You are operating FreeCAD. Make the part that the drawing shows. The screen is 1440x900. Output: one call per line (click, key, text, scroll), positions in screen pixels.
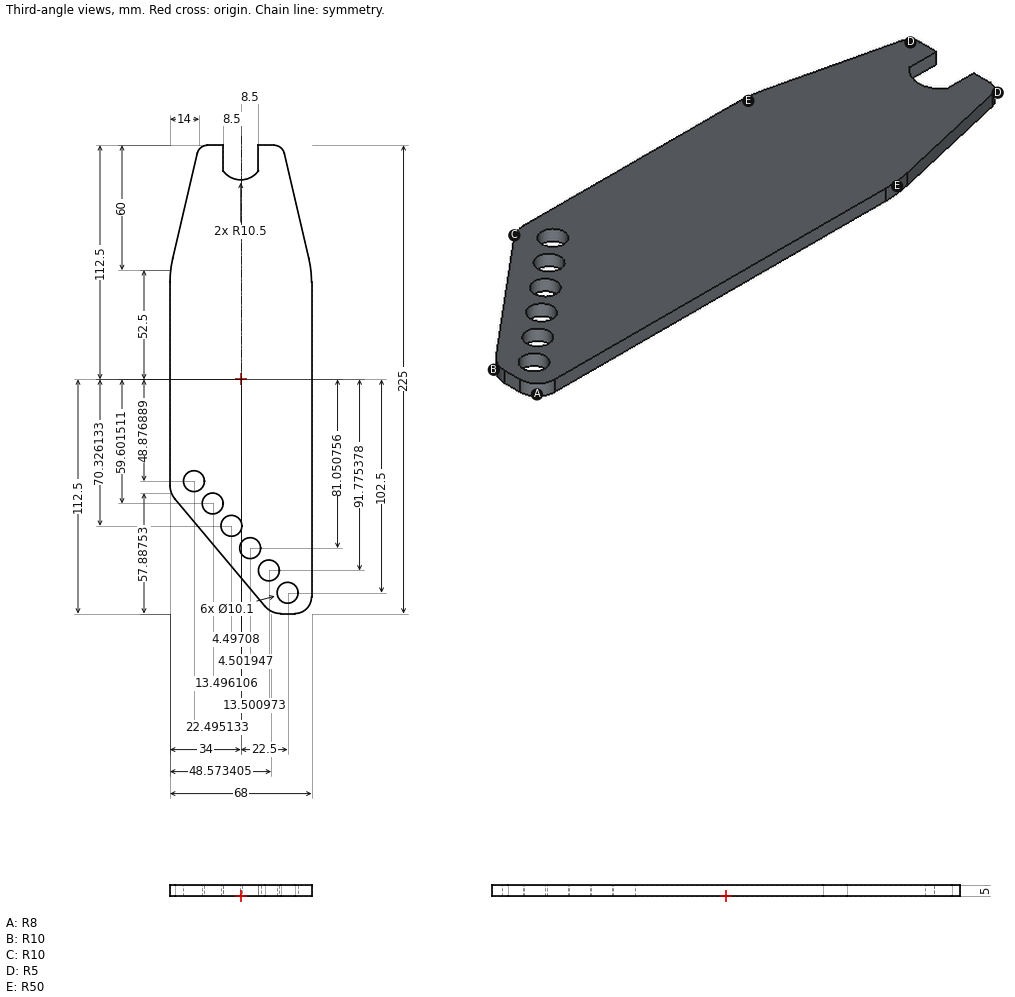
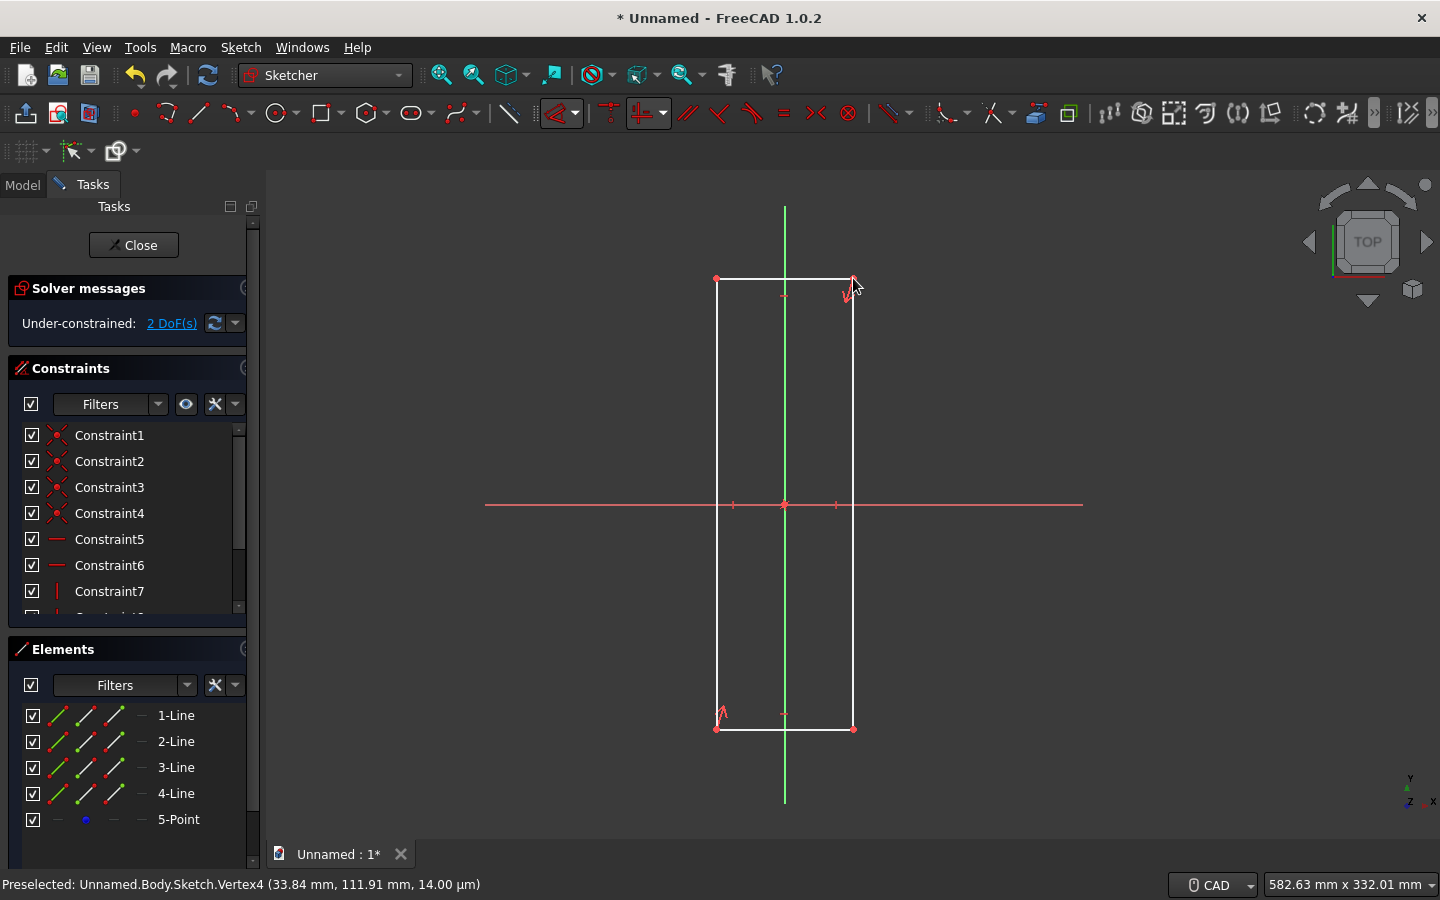
click(758, 730)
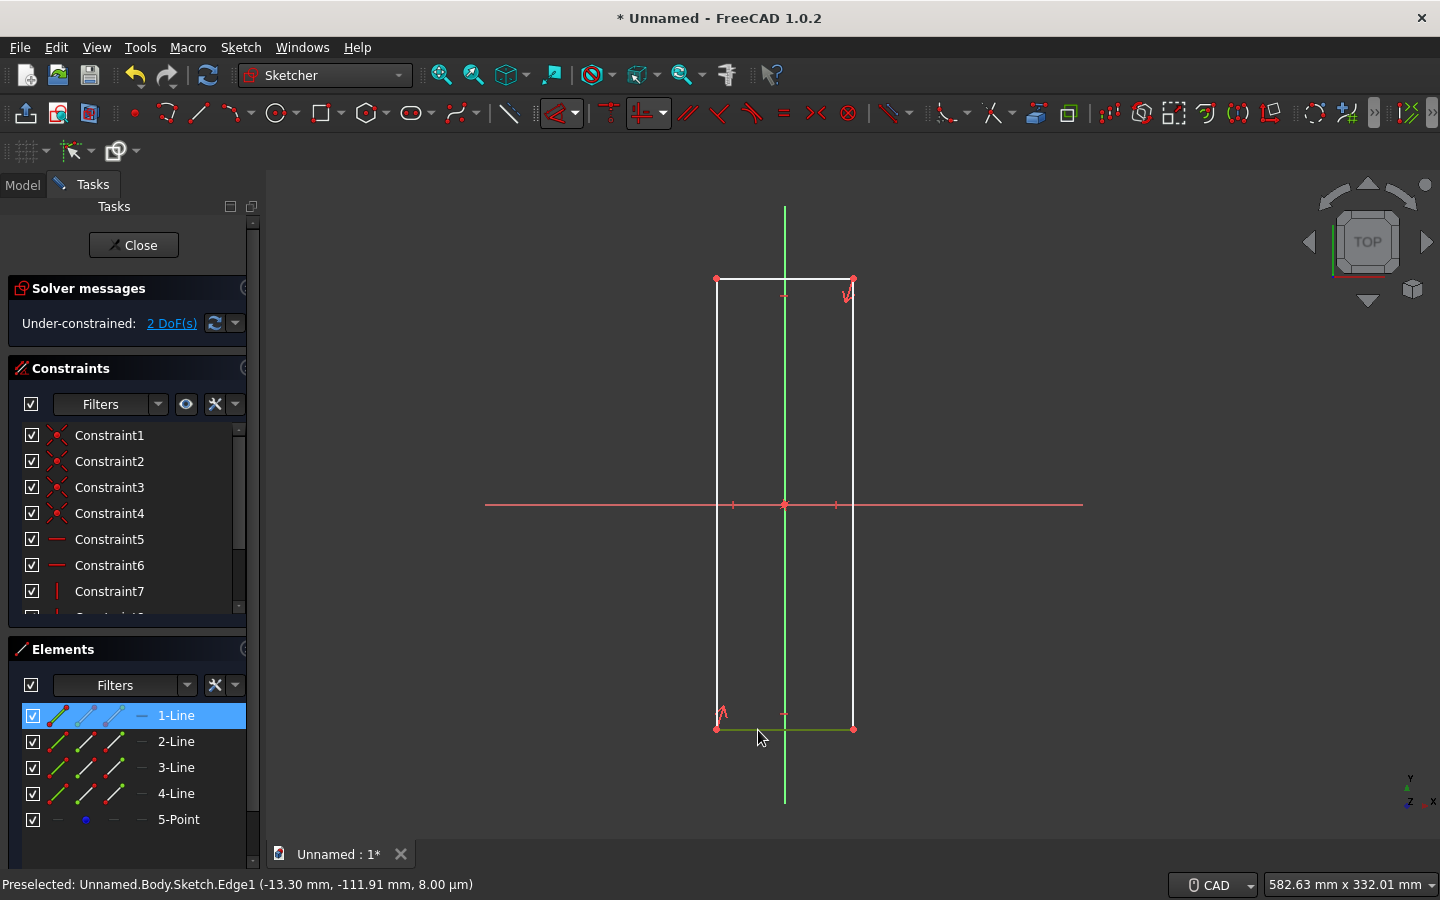
key(l)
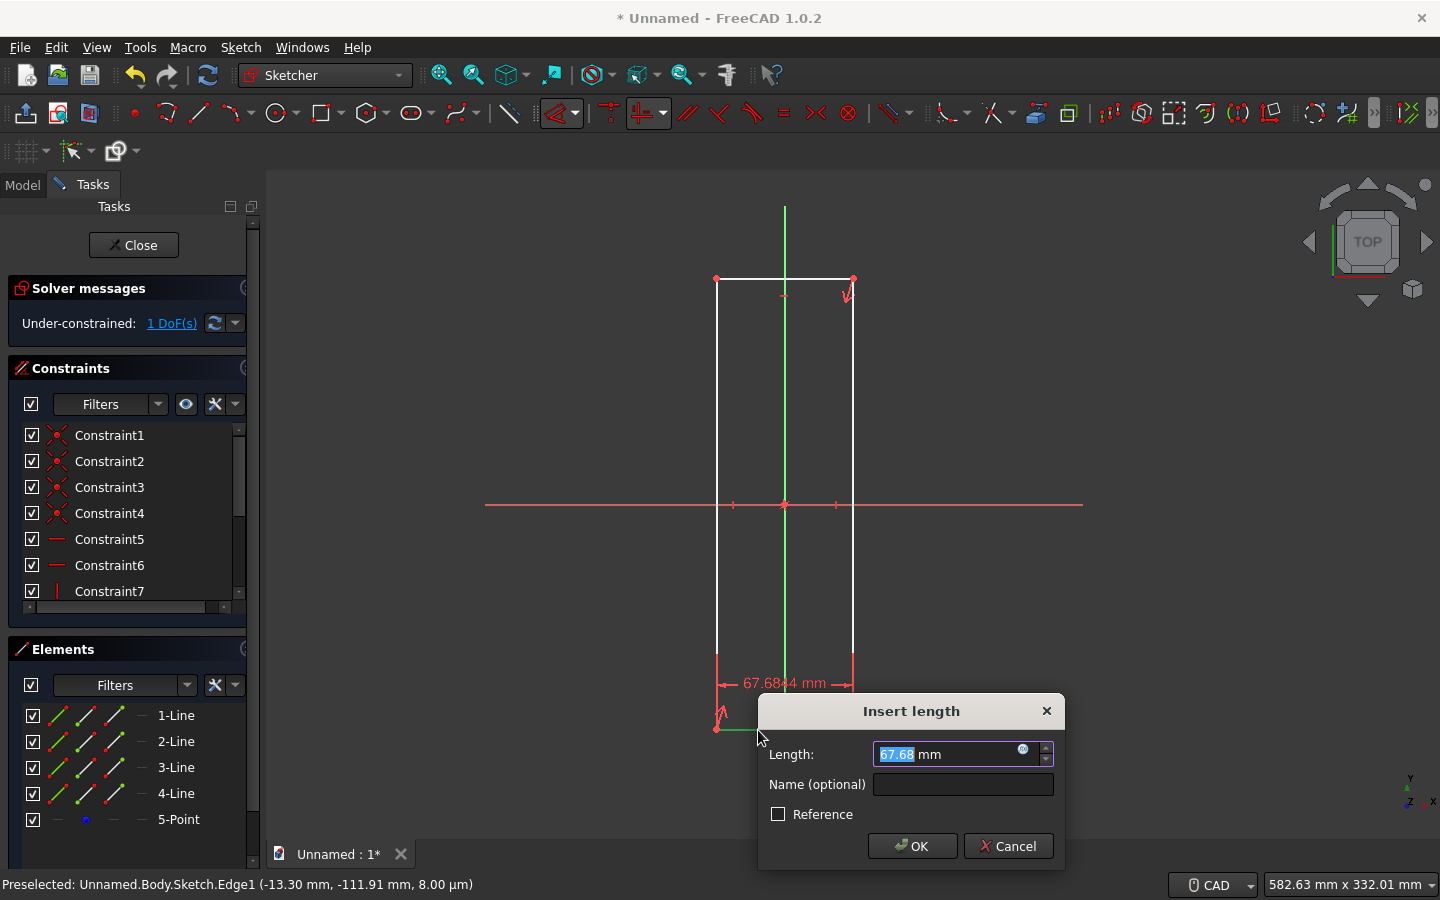
text(68)
key(Return)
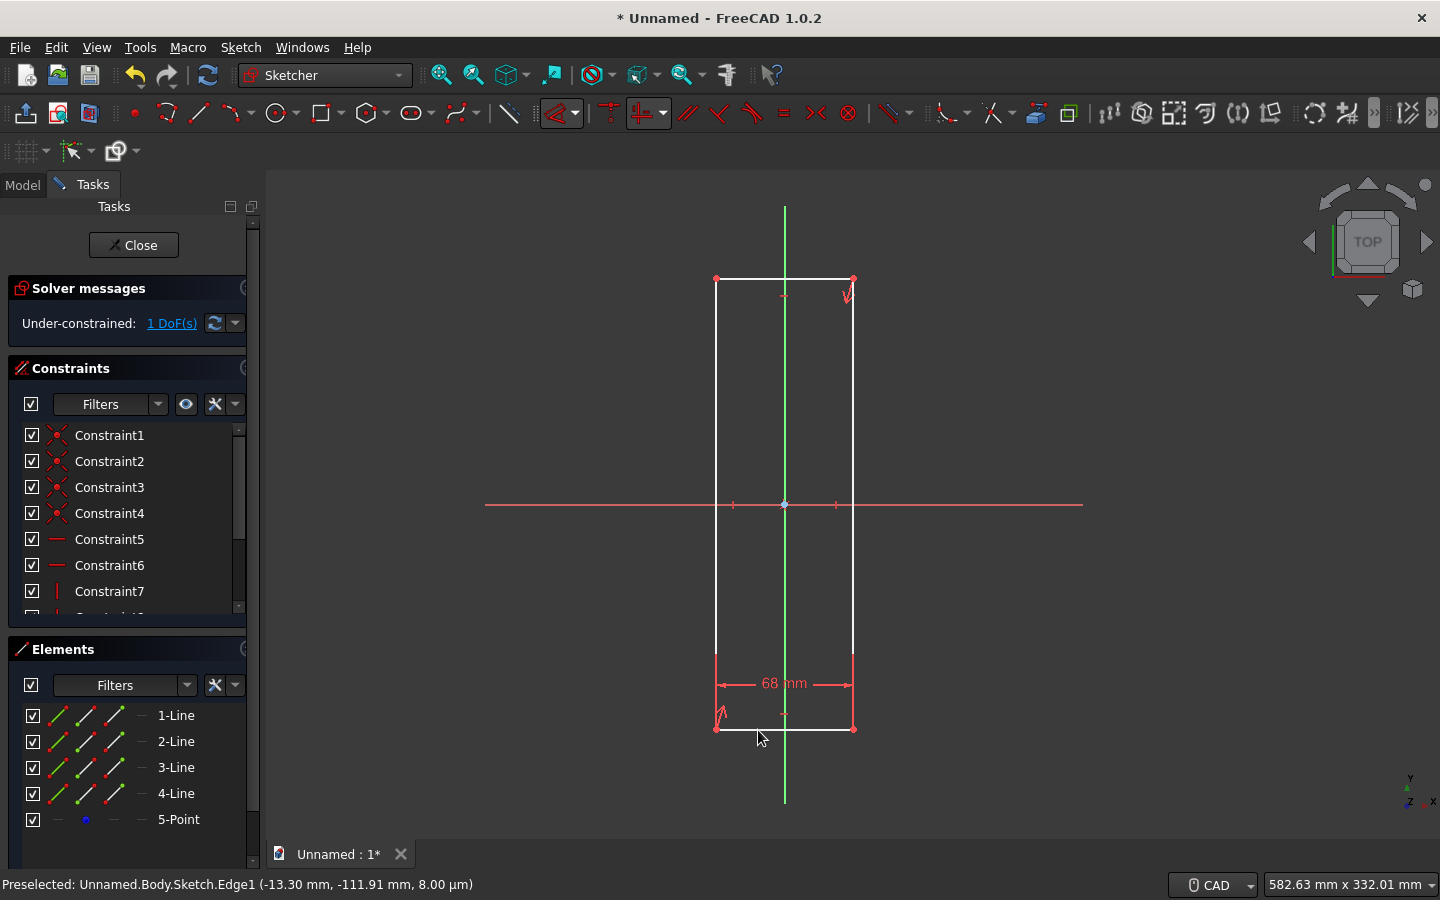
click(853, 595)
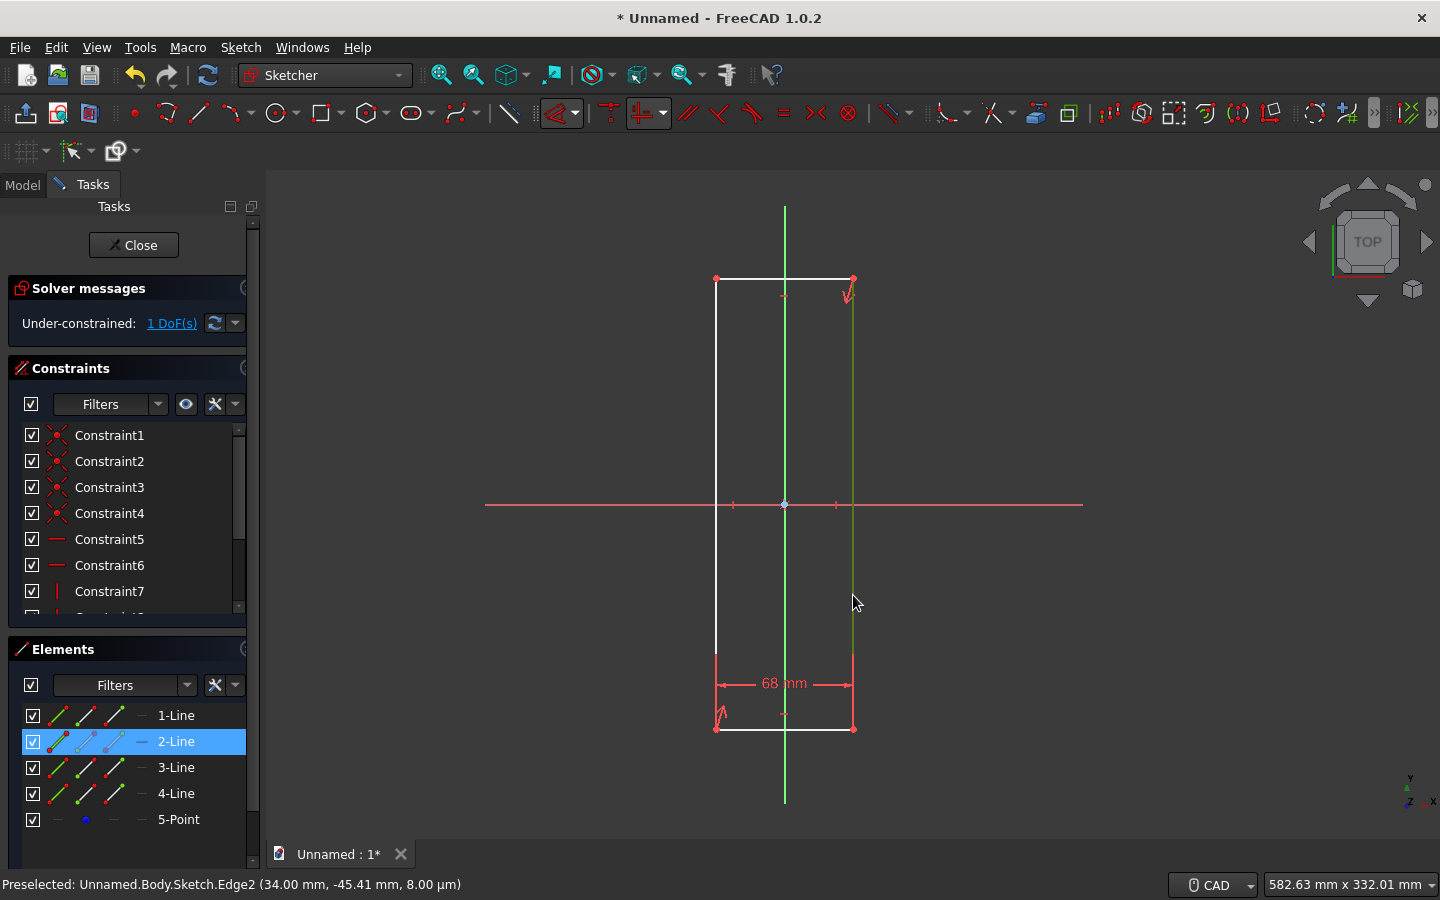
key(i)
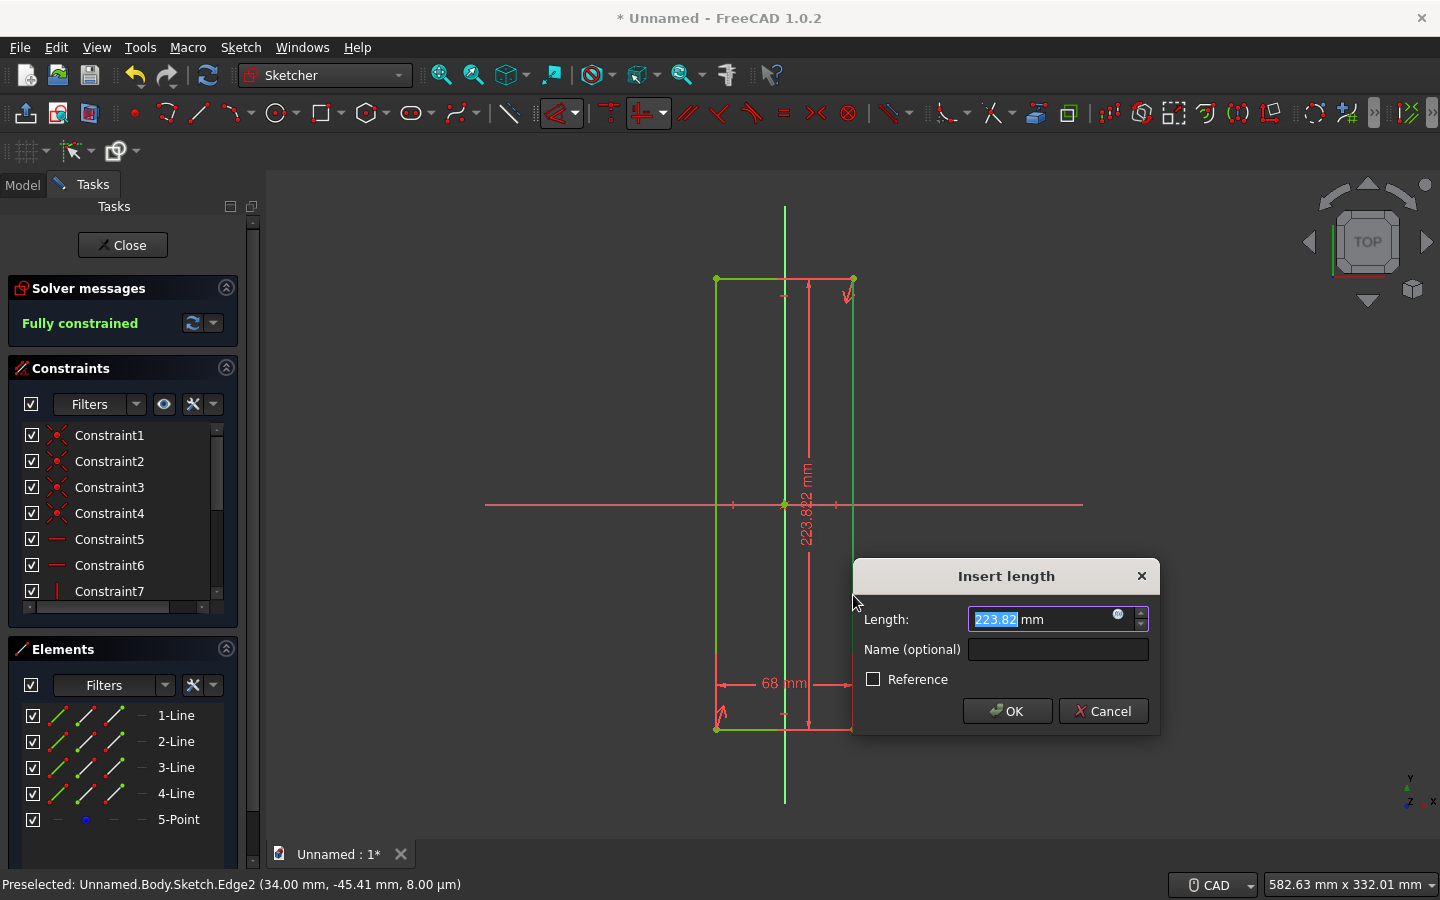
text(225)
key(Return)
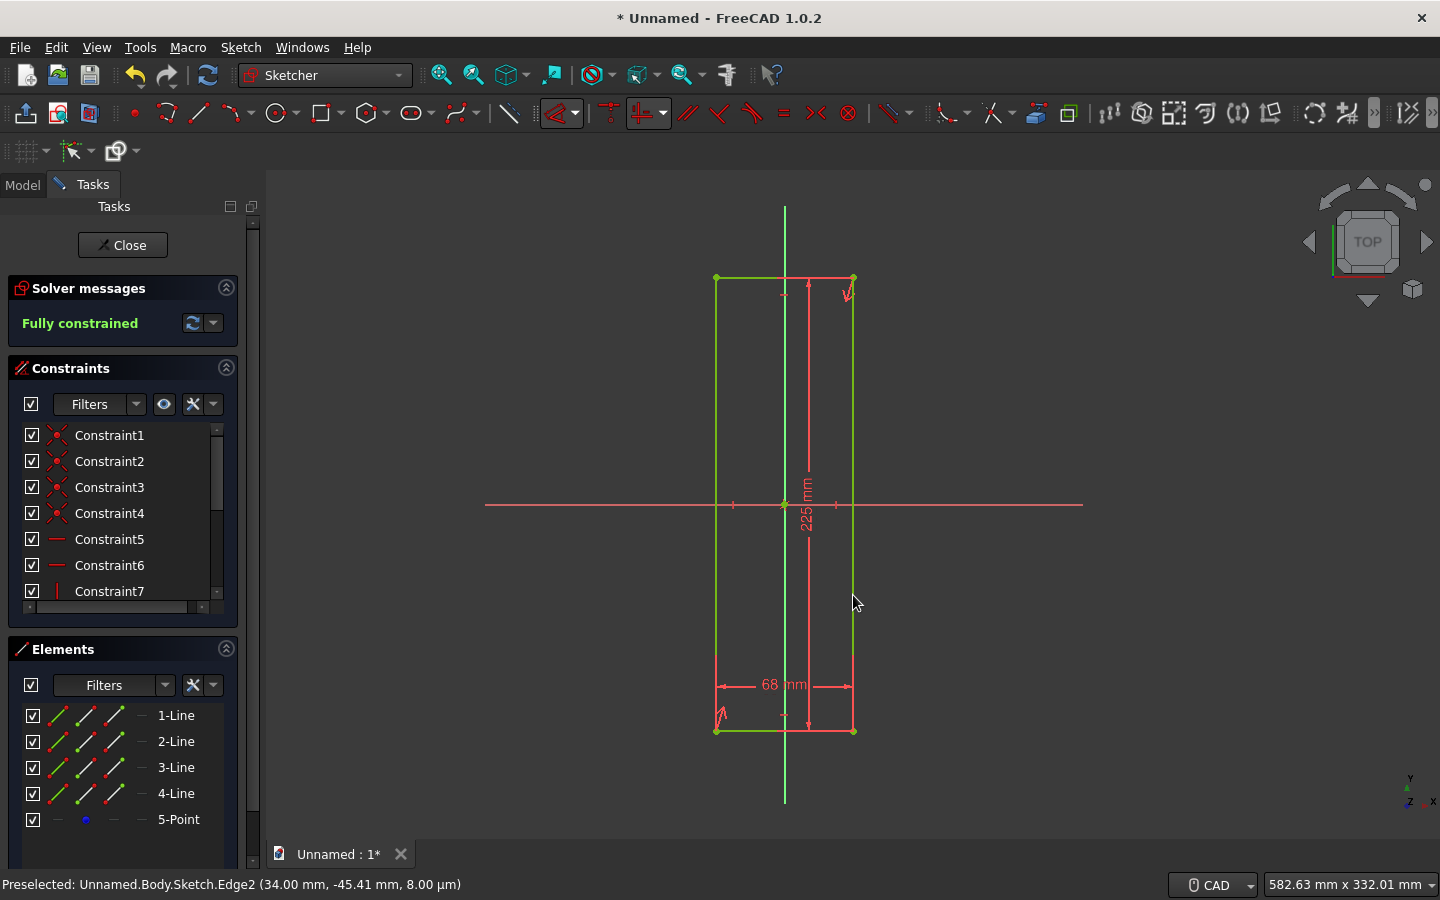
click(123, 245)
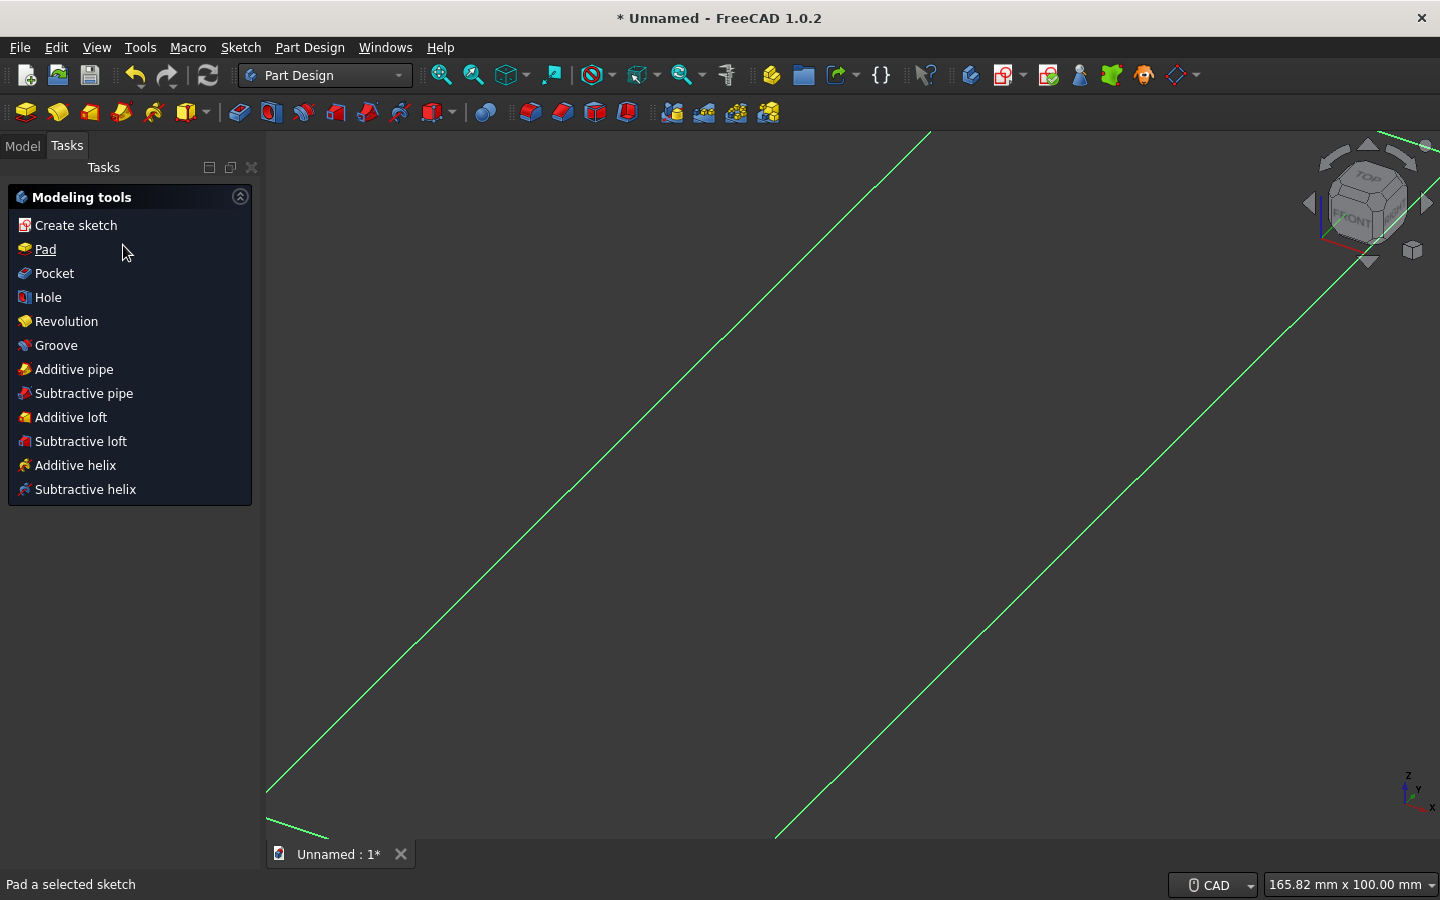
click(26, 112)